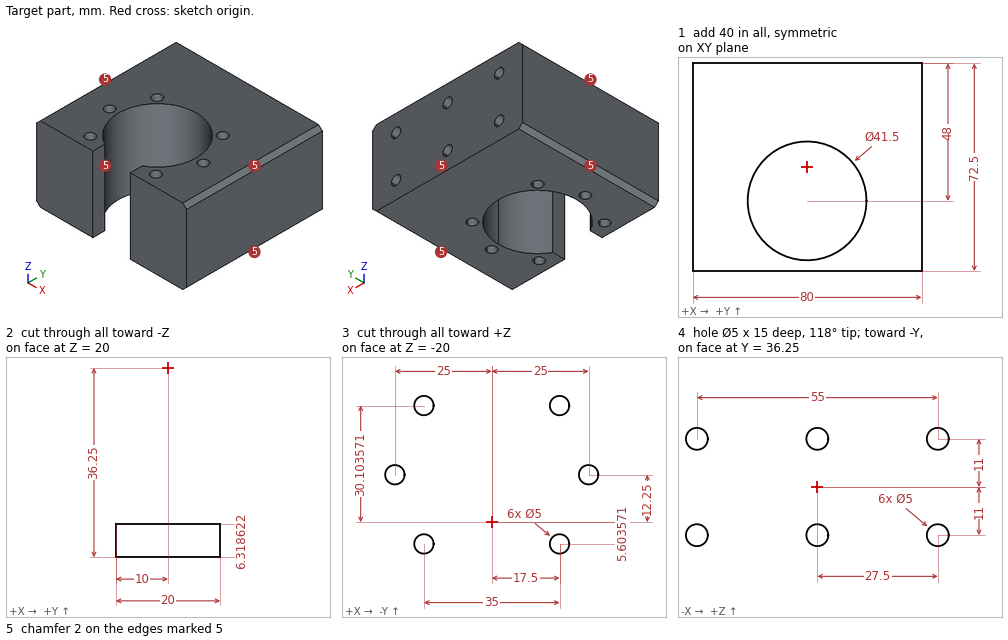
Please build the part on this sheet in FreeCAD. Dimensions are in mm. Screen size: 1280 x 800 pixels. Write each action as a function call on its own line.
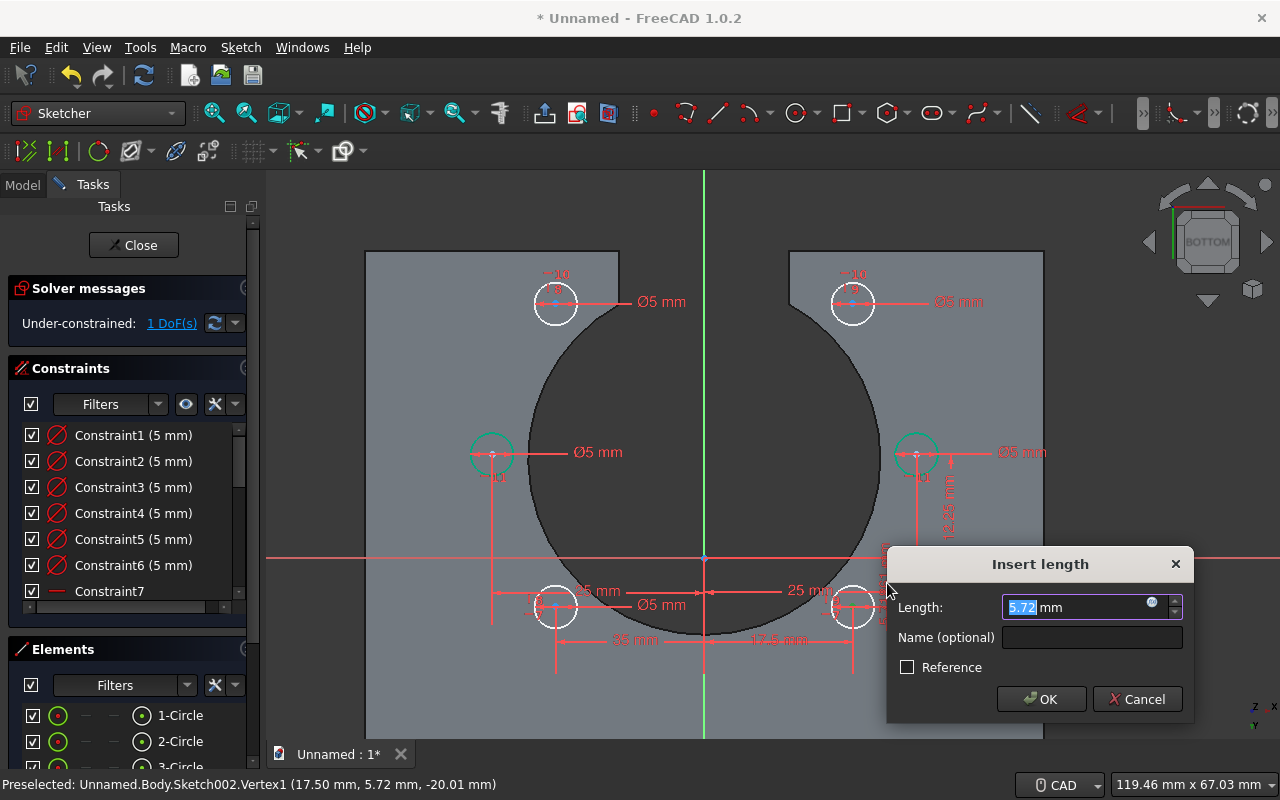
text(5.603571)
key(Return)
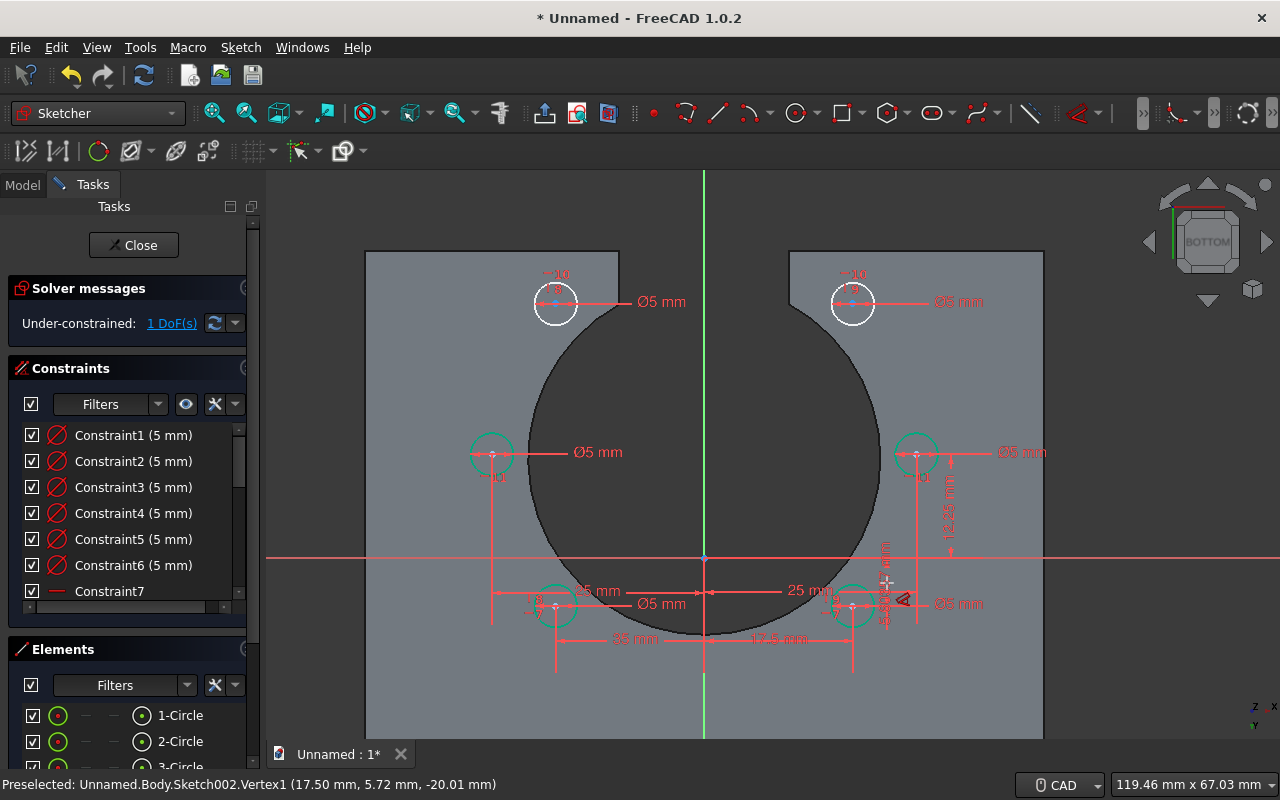
click(556, 304)
click(522, 431)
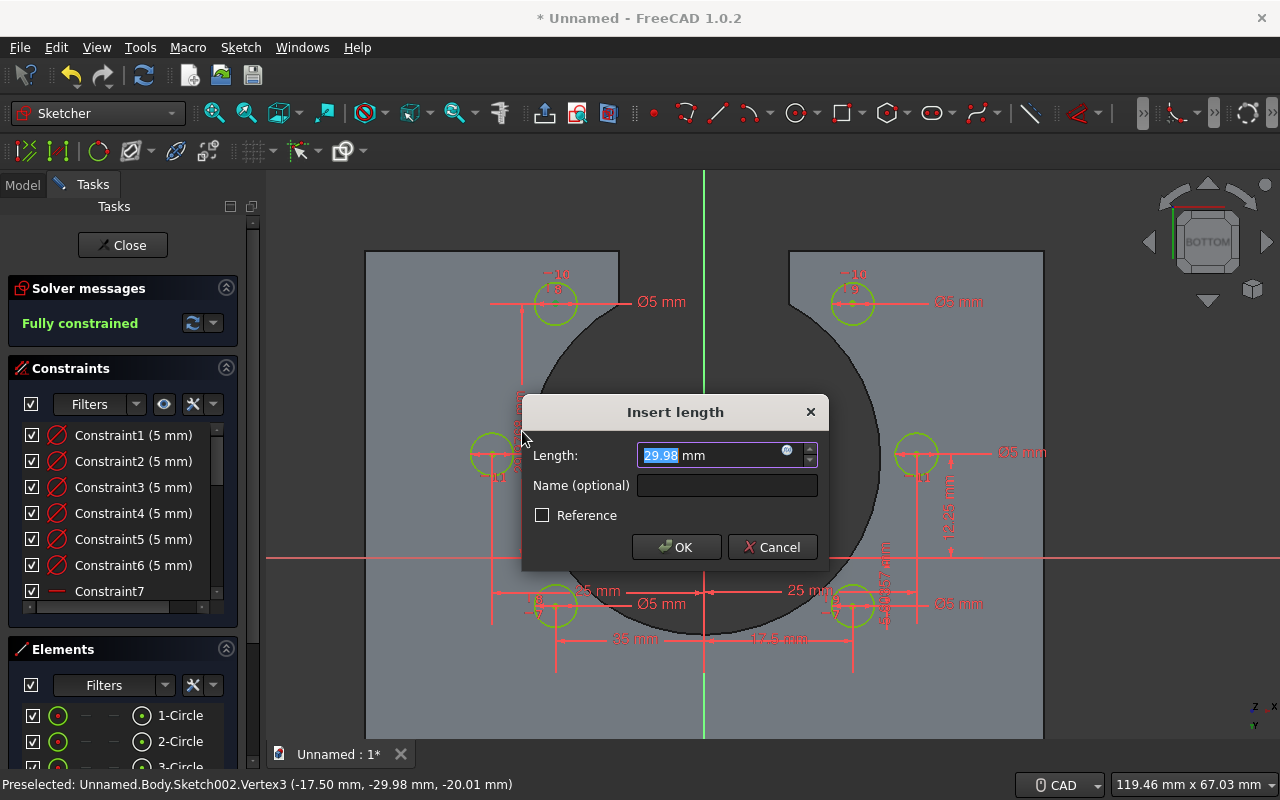
text(30.103571)
key(Return)
key(Escape)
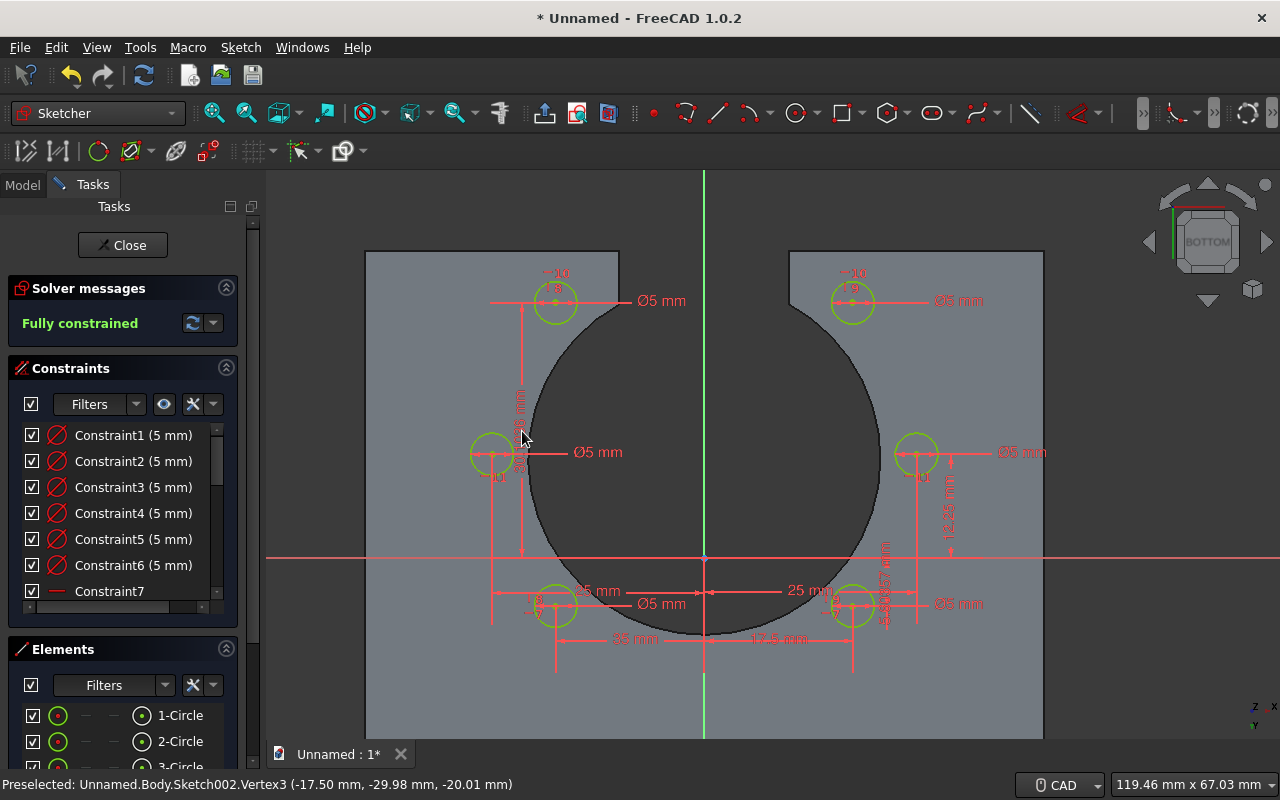
click(123, 245)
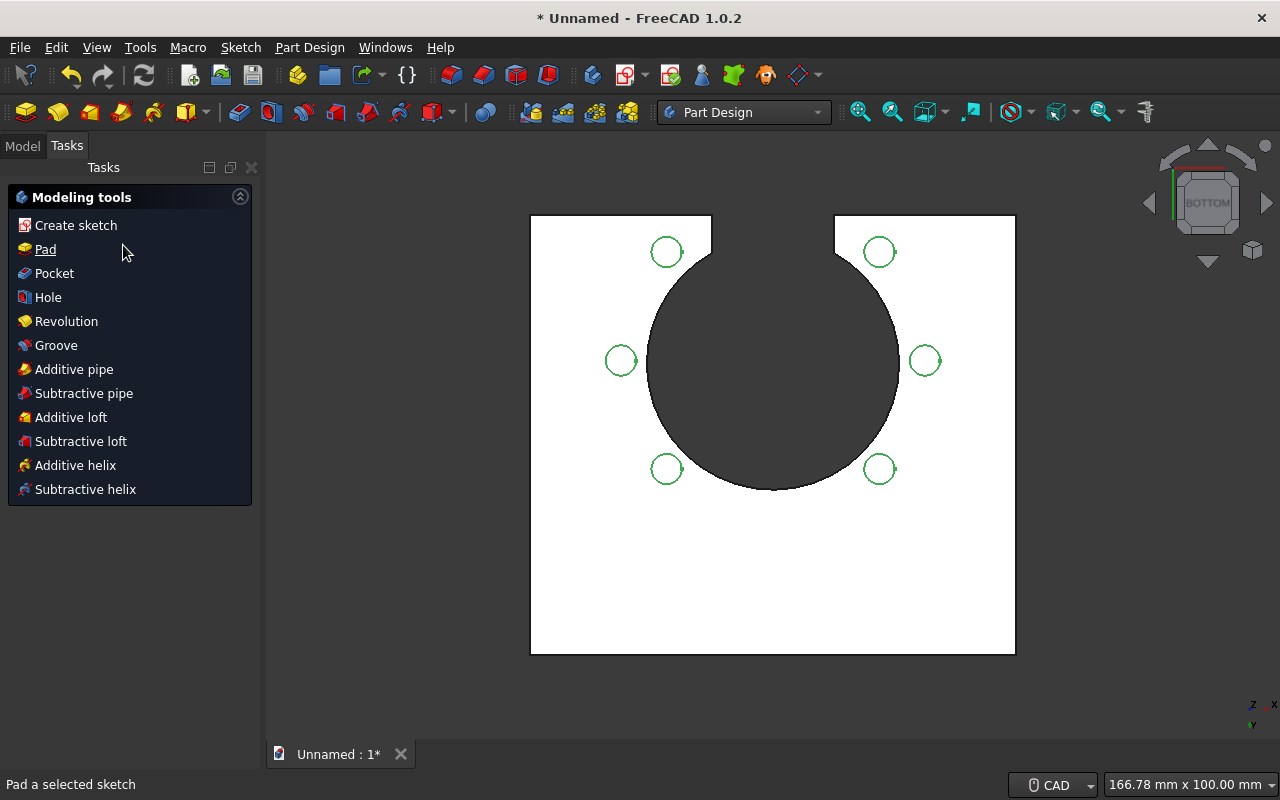
click(240, 112)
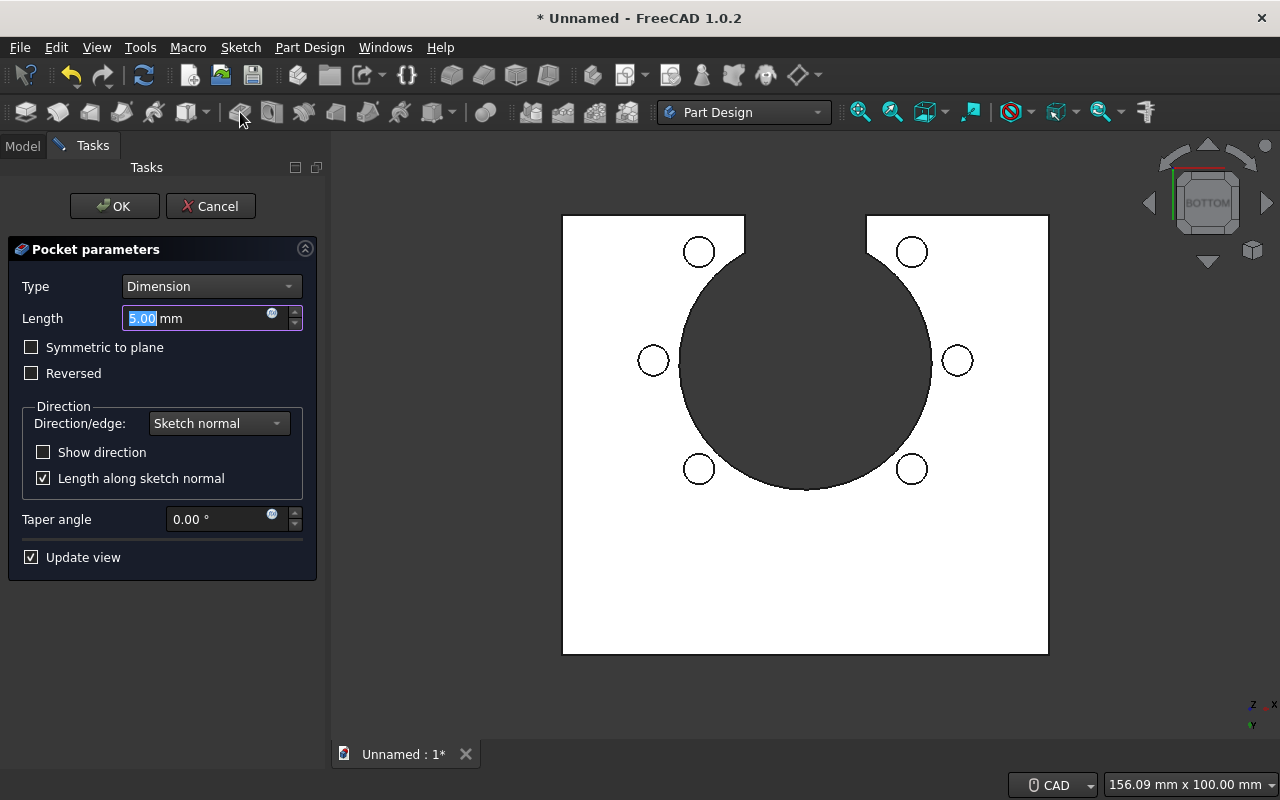
click(212, 286)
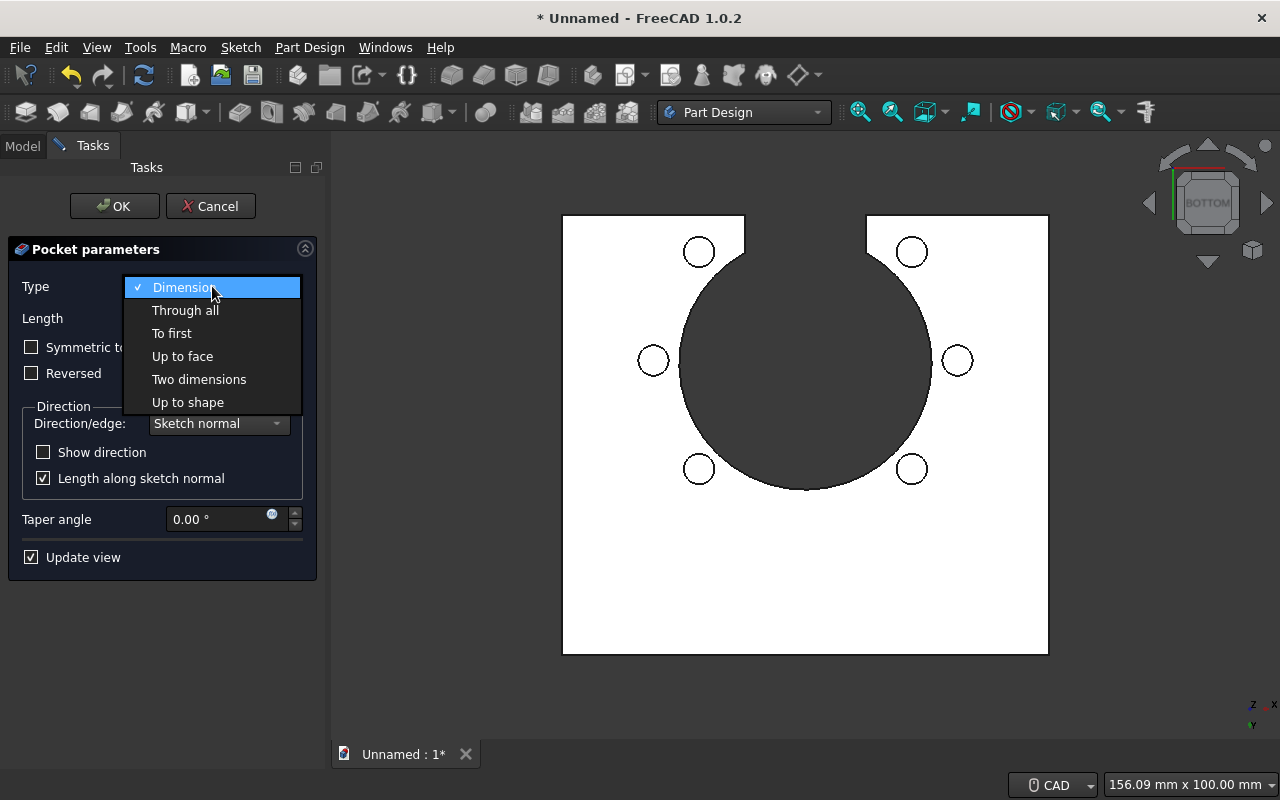
click(212, 310)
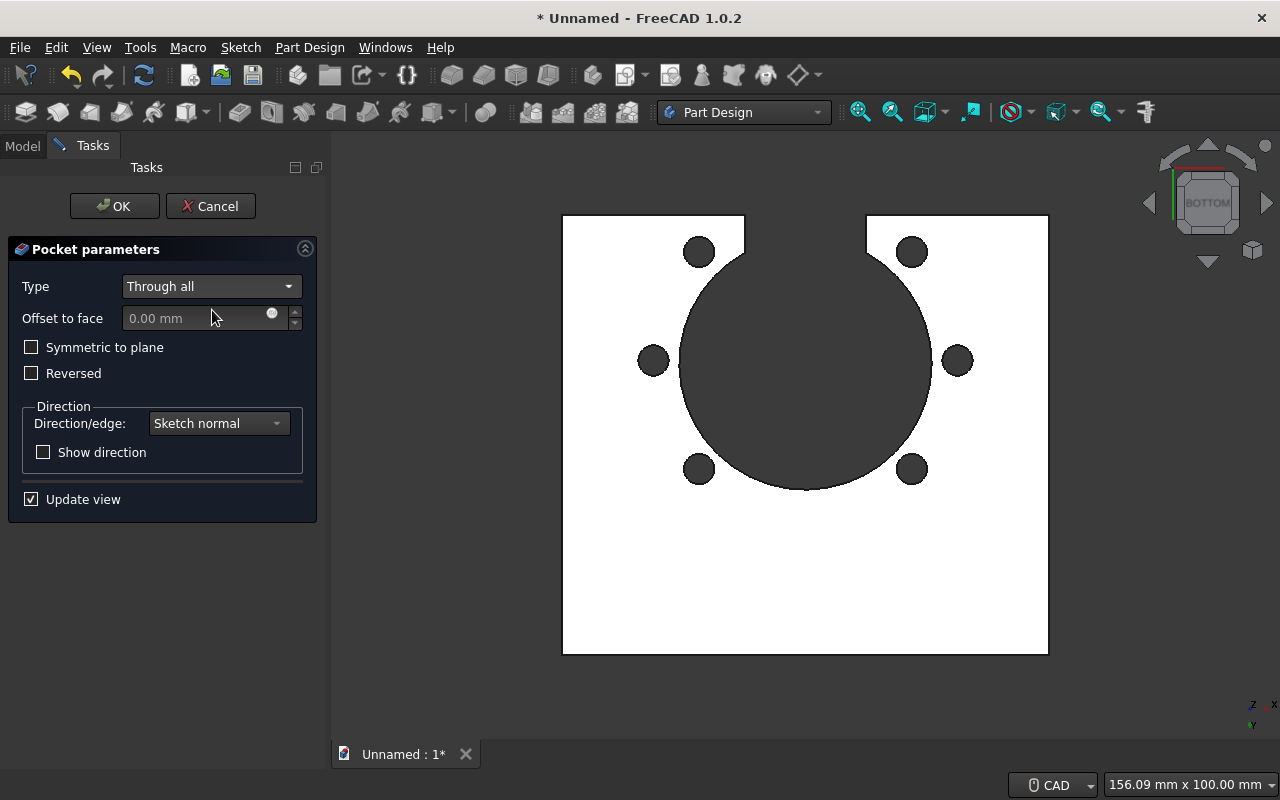
click(115, 206)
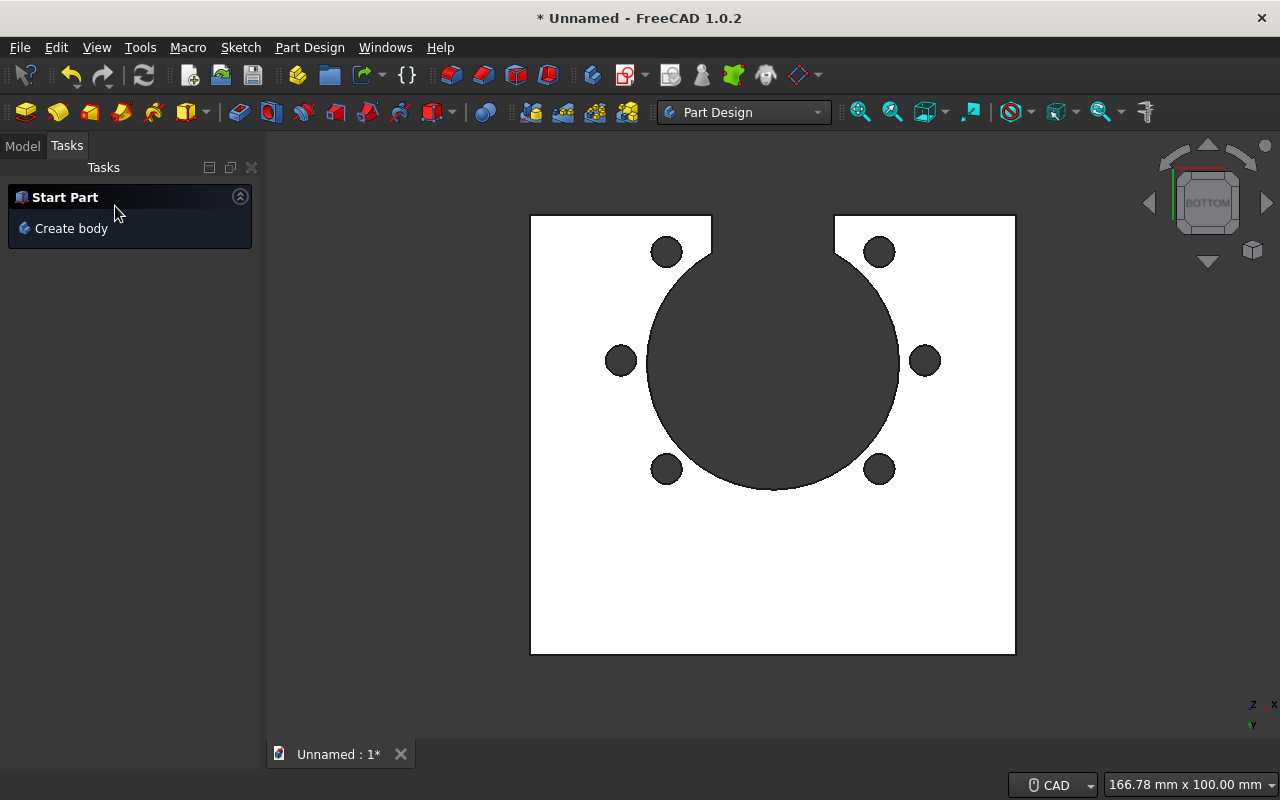
key(4)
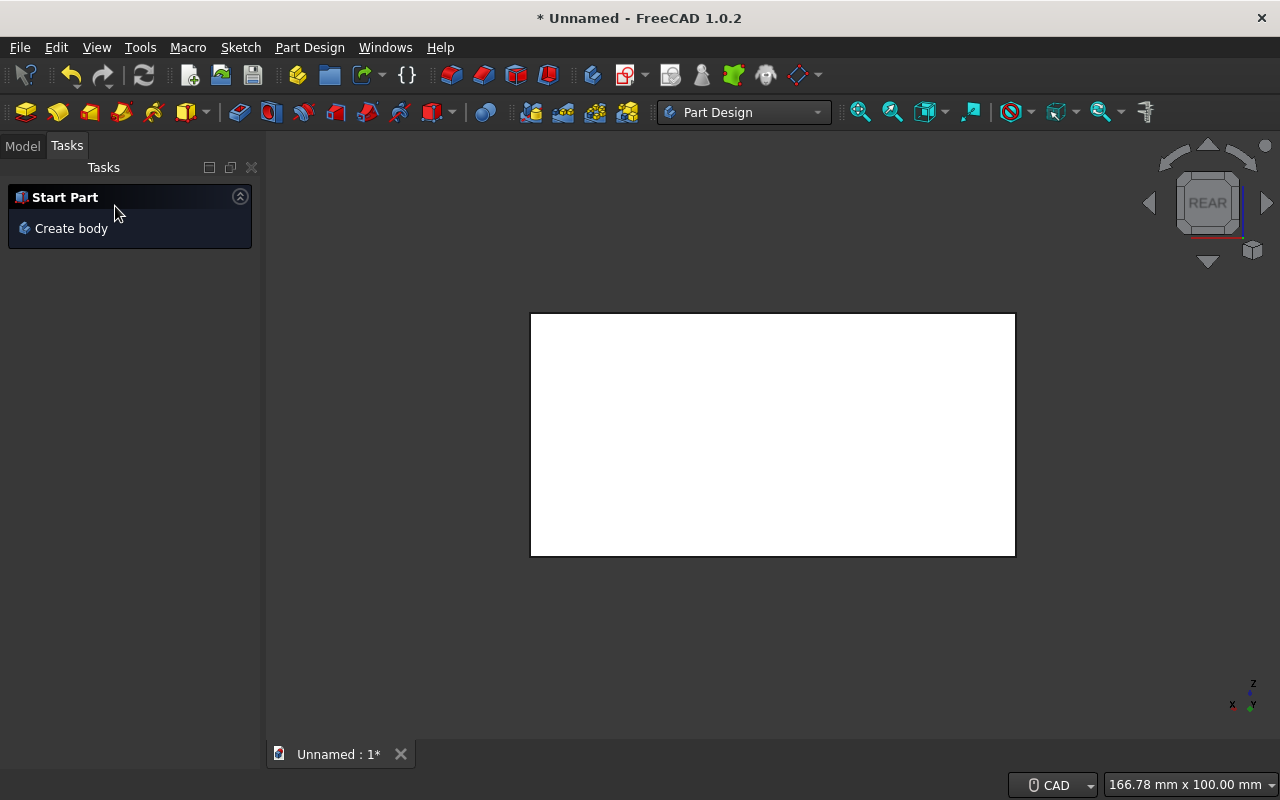
click(704, 434)